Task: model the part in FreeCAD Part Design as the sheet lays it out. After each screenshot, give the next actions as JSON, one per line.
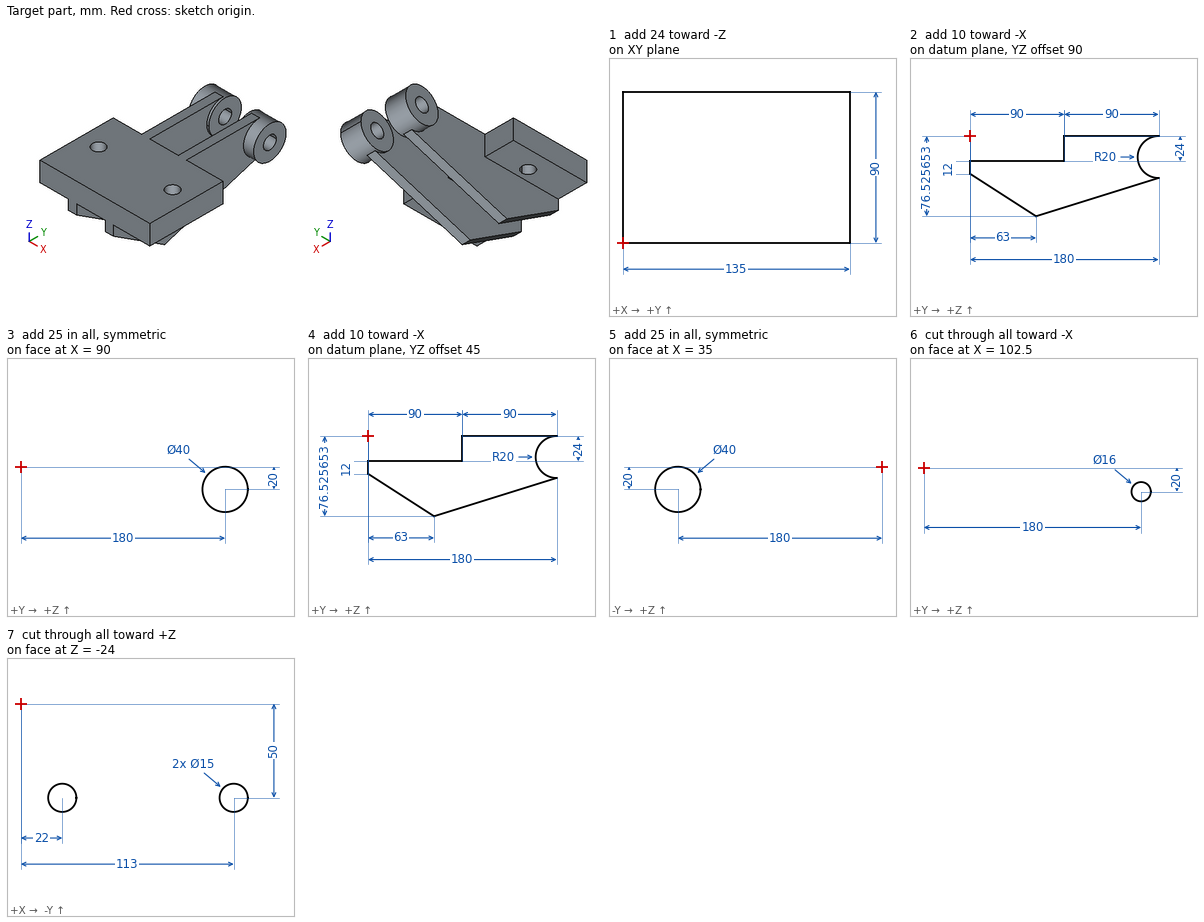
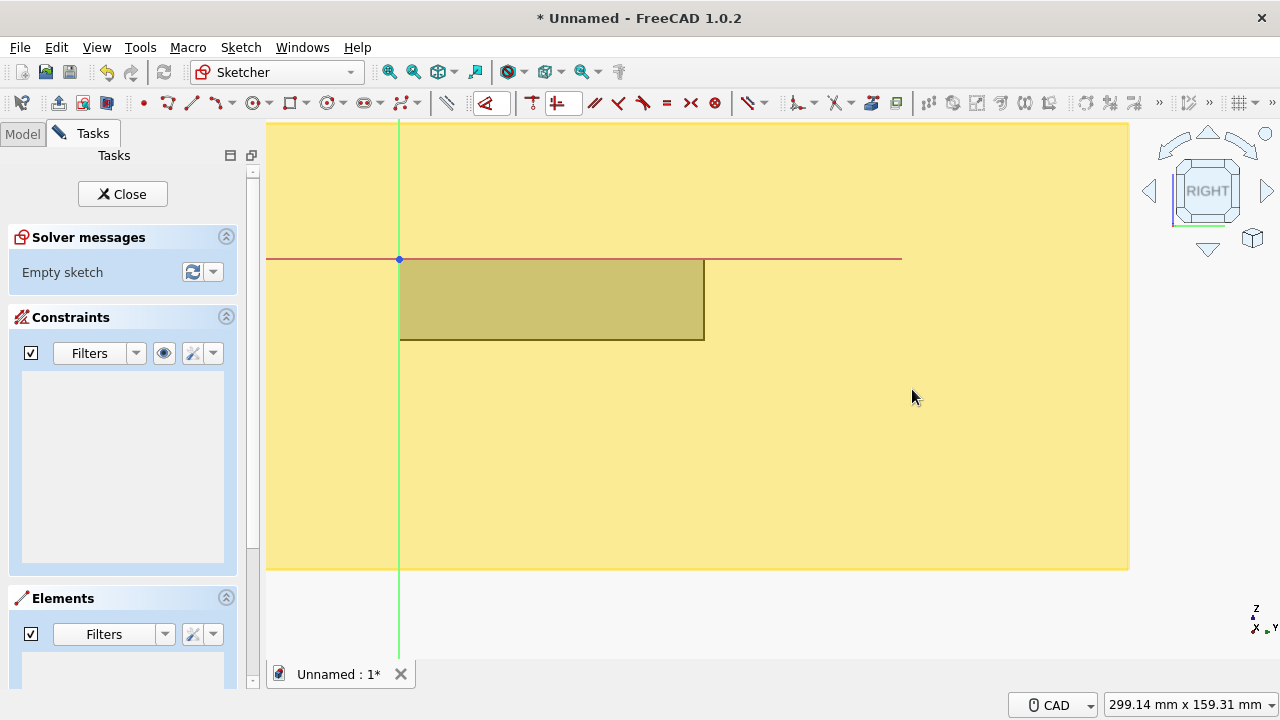
{"action": "left_click", "coordinate": [168, 104]}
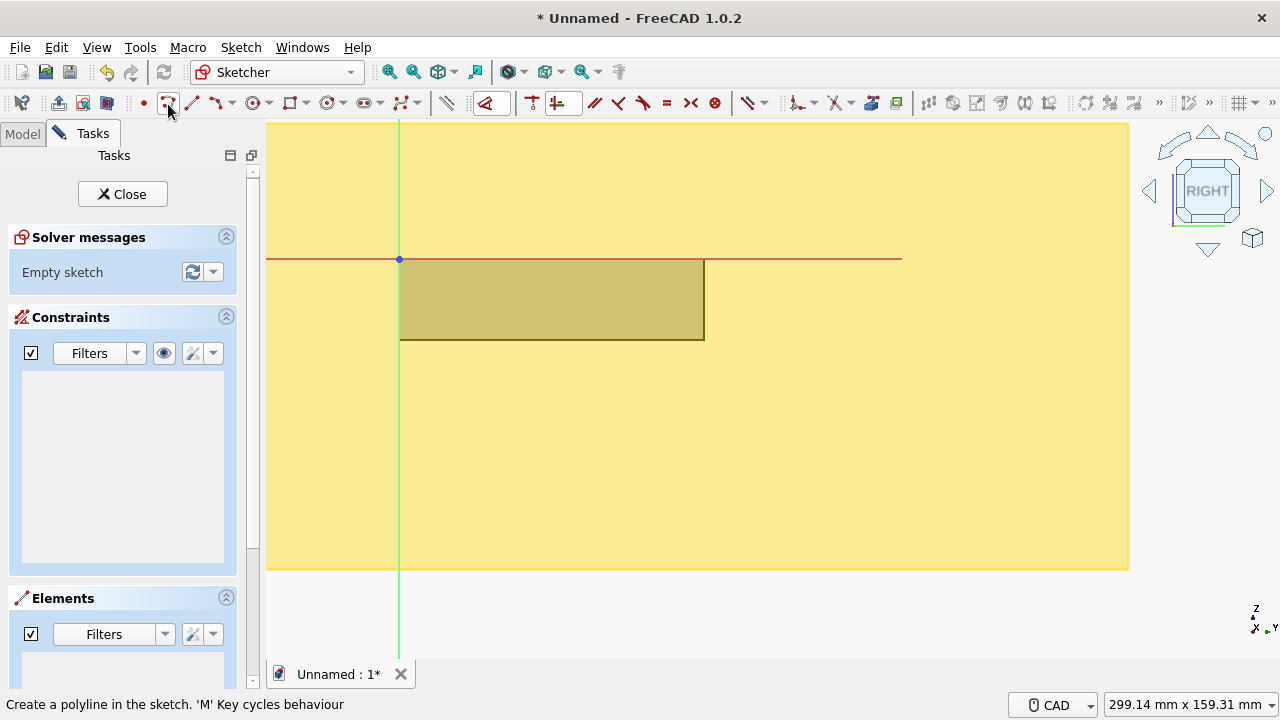
{"action": "left_click", "coordinate": [1009, 395]}
{"action": "left_click", "coordinate": [613, 518]}
{"action": "left_click", "coordinate": [399, 381]}
{"action": "left_click", "coordinate": [408, 340]}
{"action": "left_click", "coordinate": [704, 340]}
{"action": "left_click", "coordinate": [704, 259]}
{"action": "left_click", "coordinate": [1009, 268]}
{"action": "right_click", "coordinate": [1009, 268]}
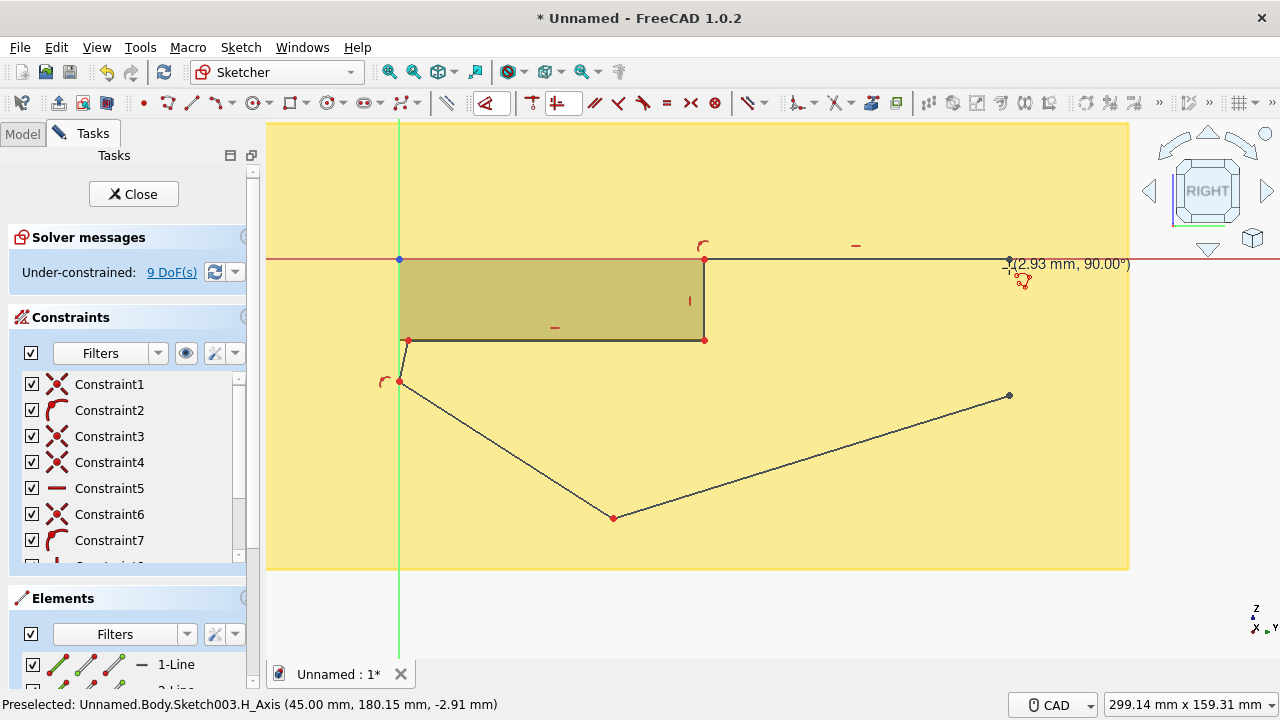
{"action": "left_click", "coordinate": [216, 104]}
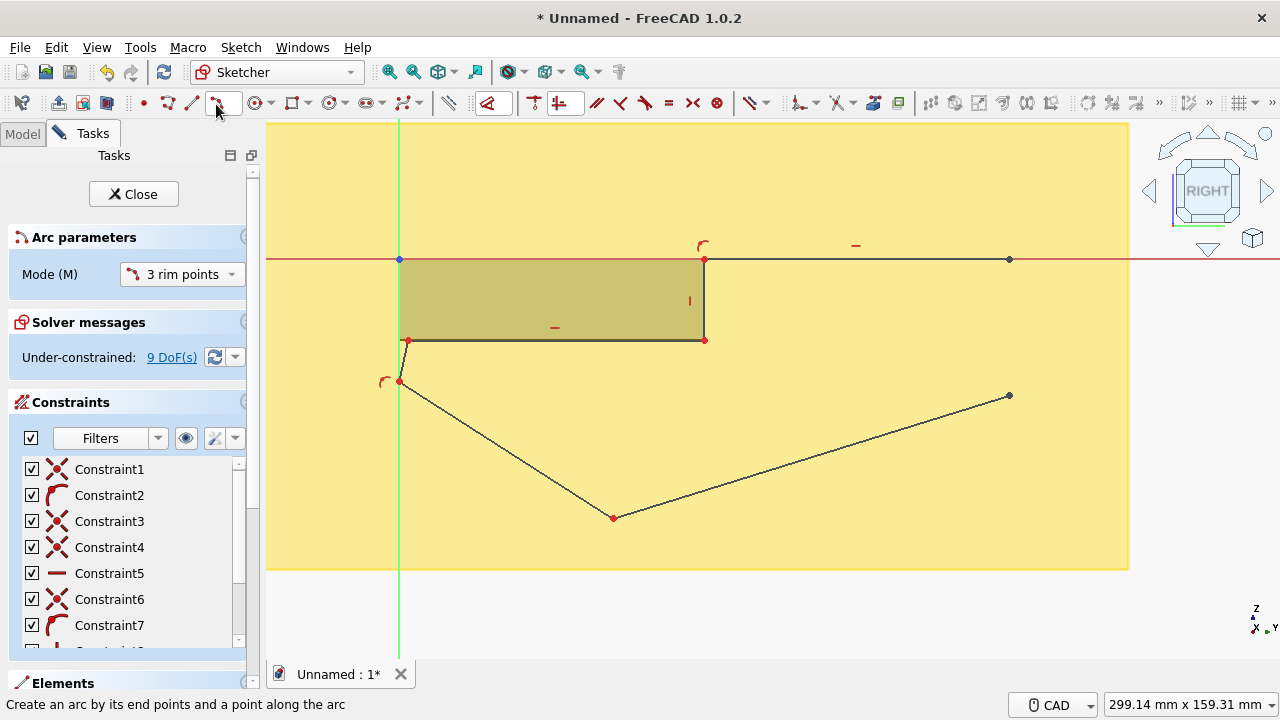
{"action": "left_click", "coordinate": [1009, 259]}
{"action": "left_click", "coordinate": [1009, 396]}
{"action": "left_click", "coordinate": [942, 327]}
{"action": "key", "text": "Escape"}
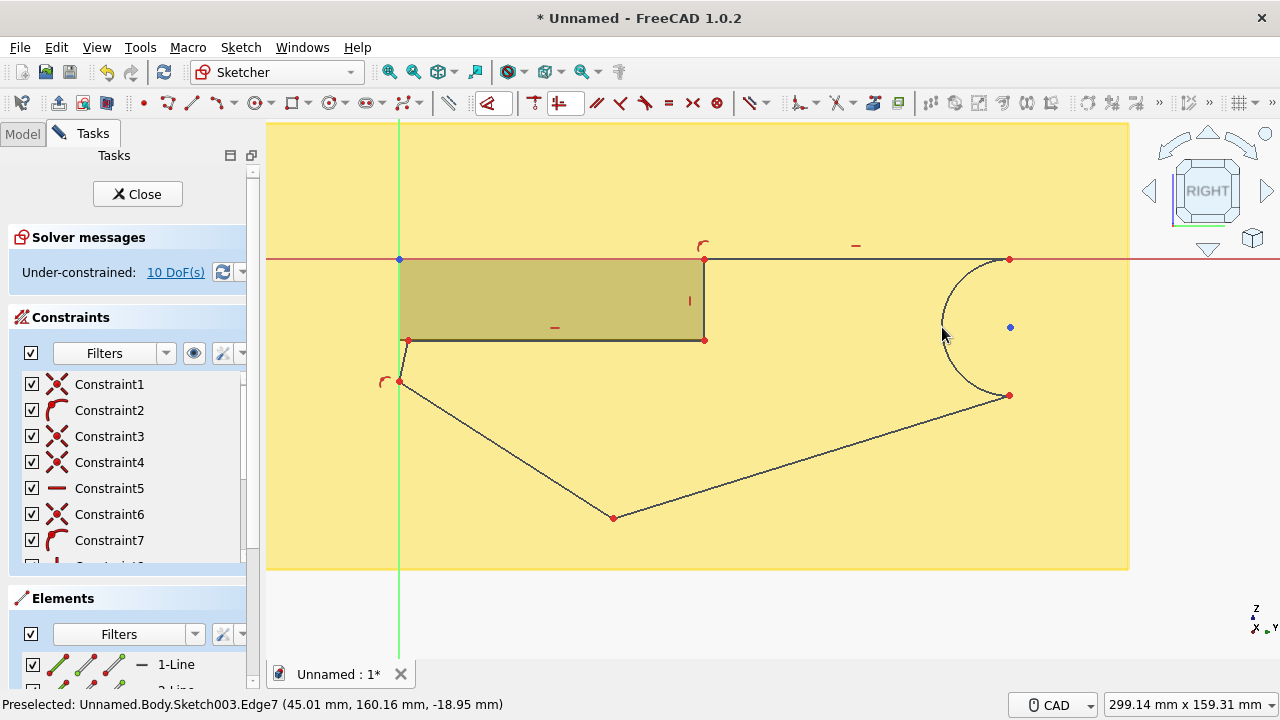
{"action": "left_click", "coordinate": [795, 259]}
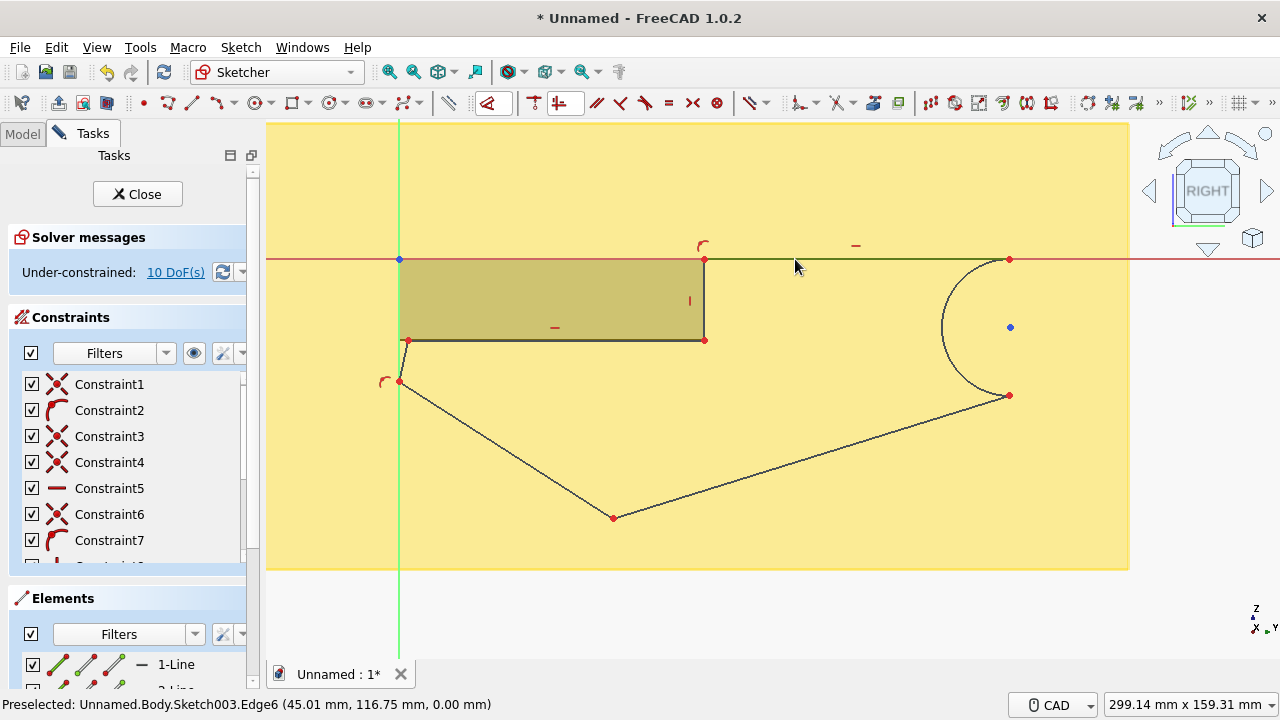
{"action": "left_click", "coordinate": [955, 288]}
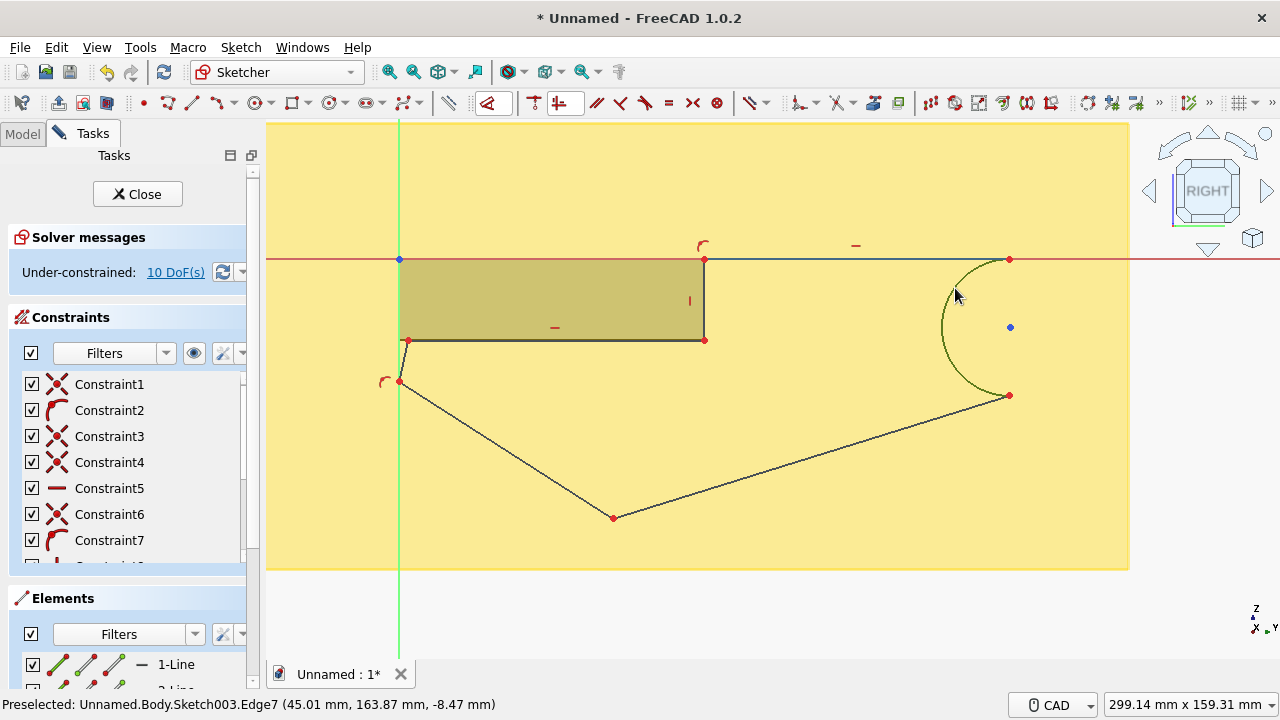
{"action": "left_click", "coordinate": [646, 104]}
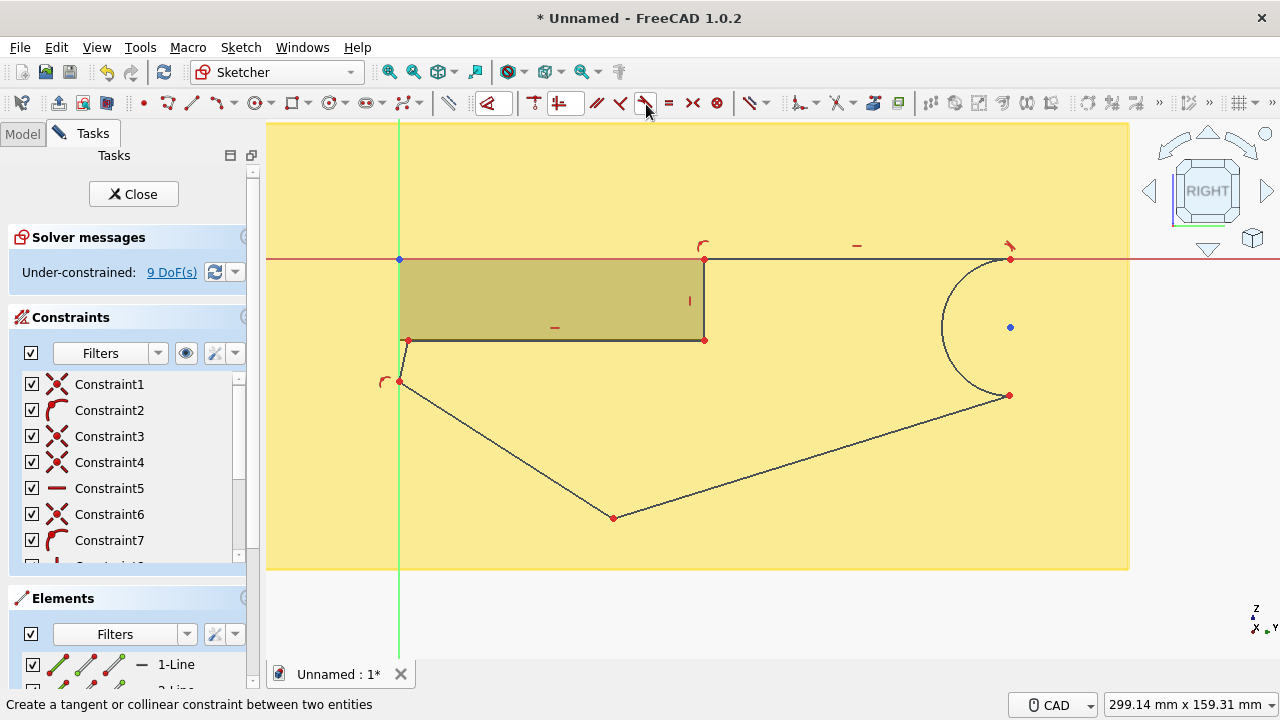
{"action": "left_click", "coordinate": [402, 370]}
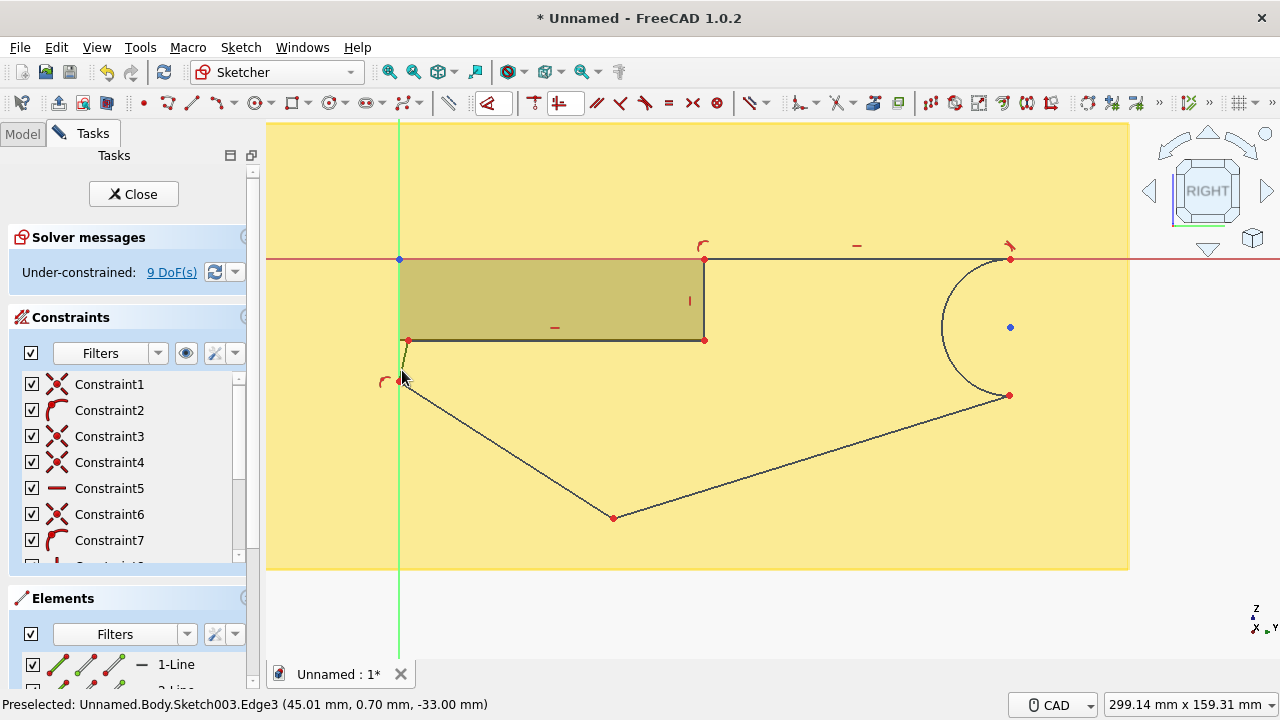
{"action": "left_click", "coordinate": [578, 104]}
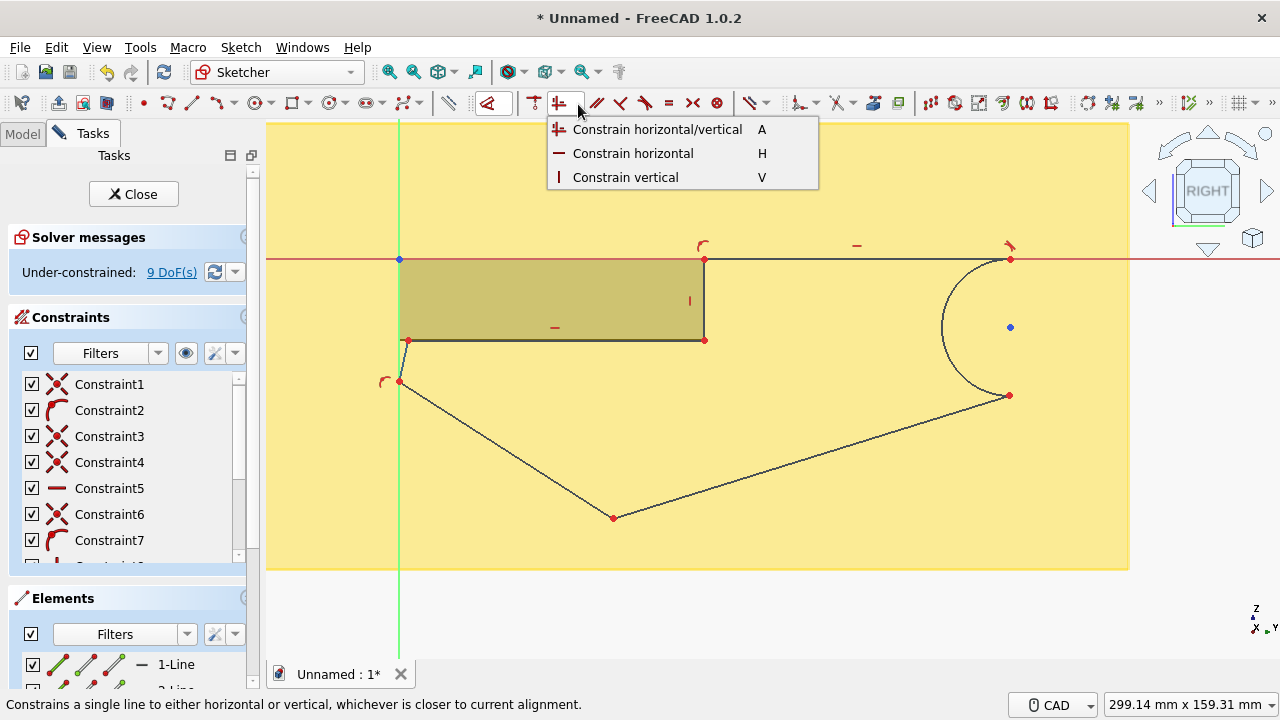
{"action": "left_click", "coordinate": [683, 177]}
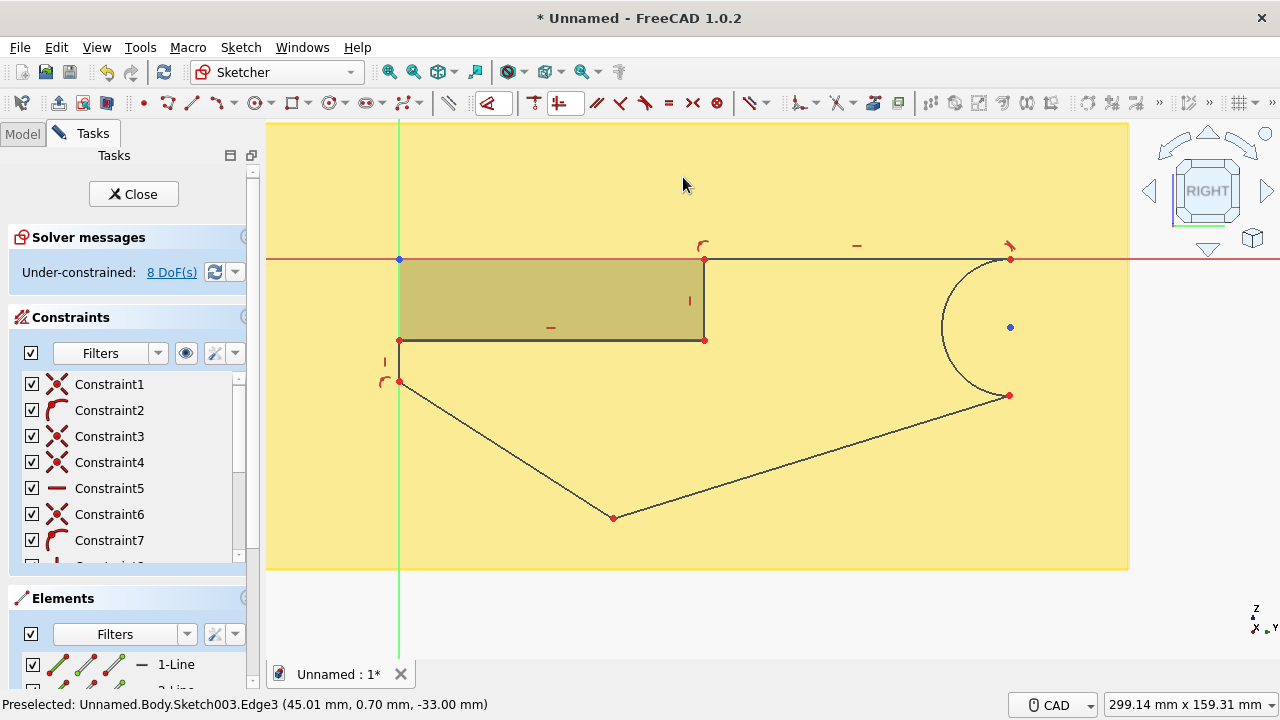
{"action": "left_click", "coordinate": [955, 287]}